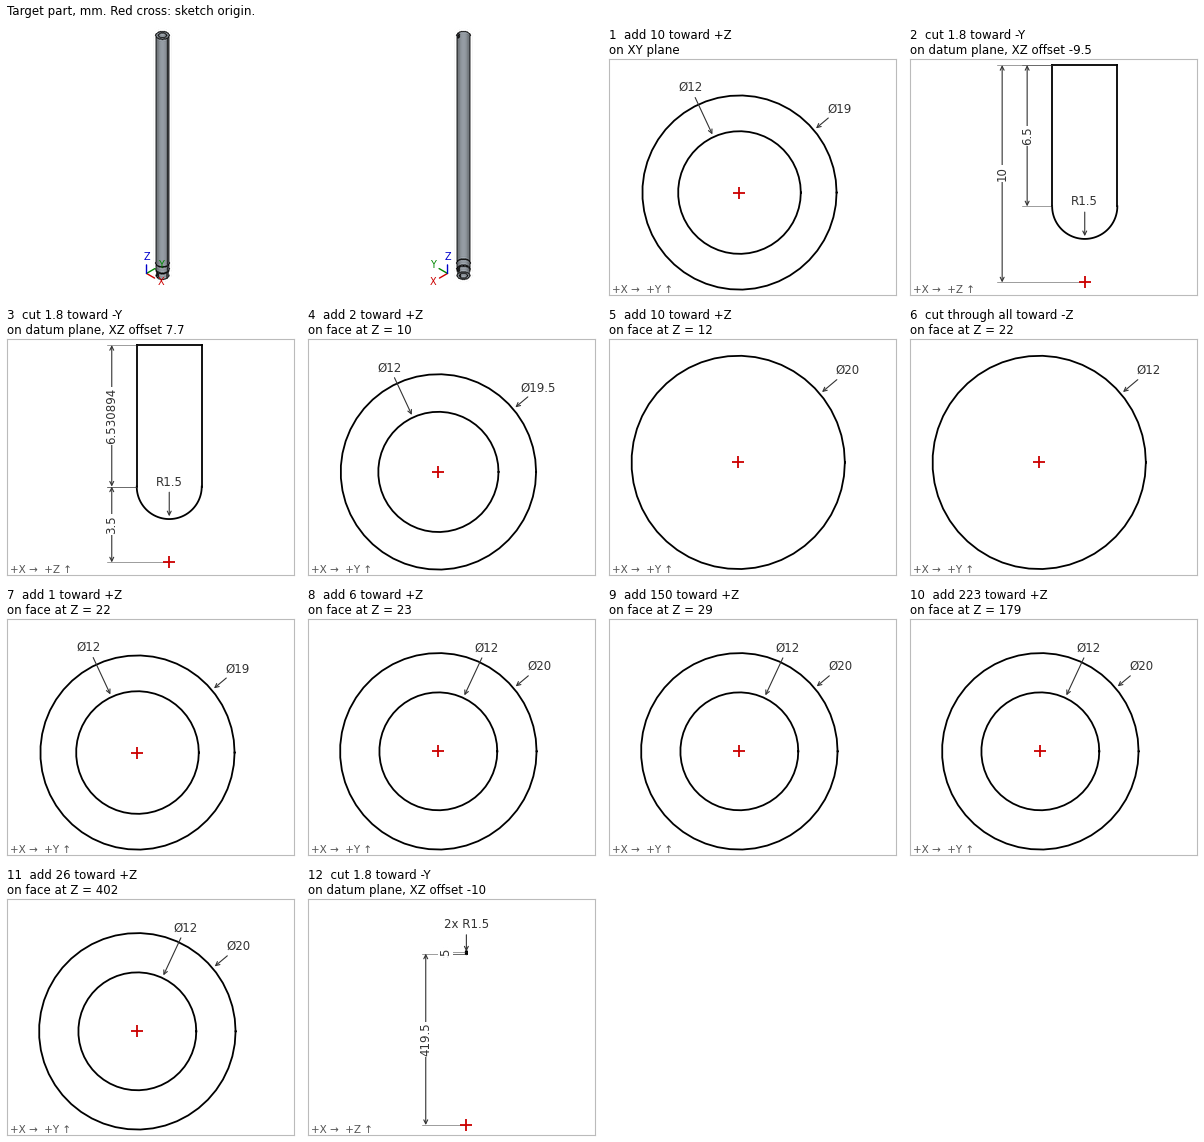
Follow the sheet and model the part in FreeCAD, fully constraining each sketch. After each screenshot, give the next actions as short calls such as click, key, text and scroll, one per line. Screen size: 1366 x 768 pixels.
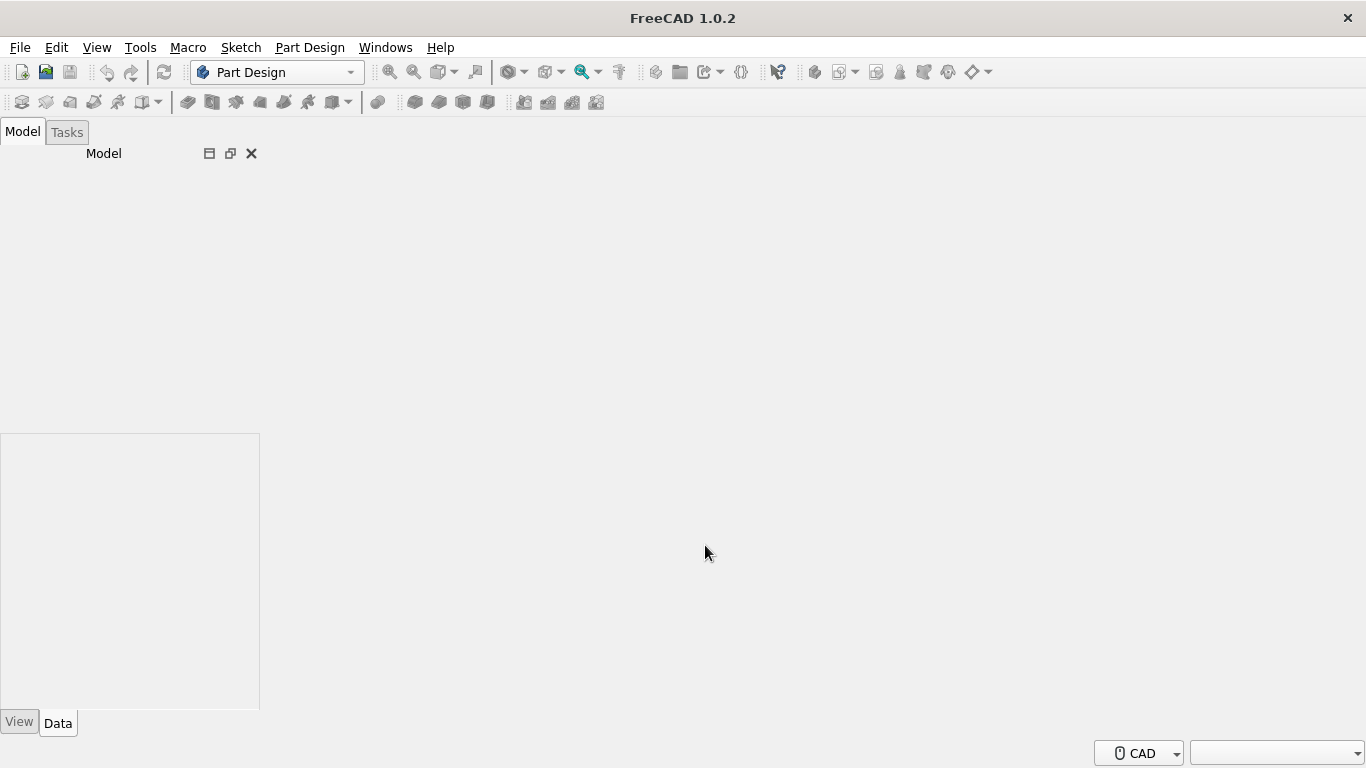
click(22, 72)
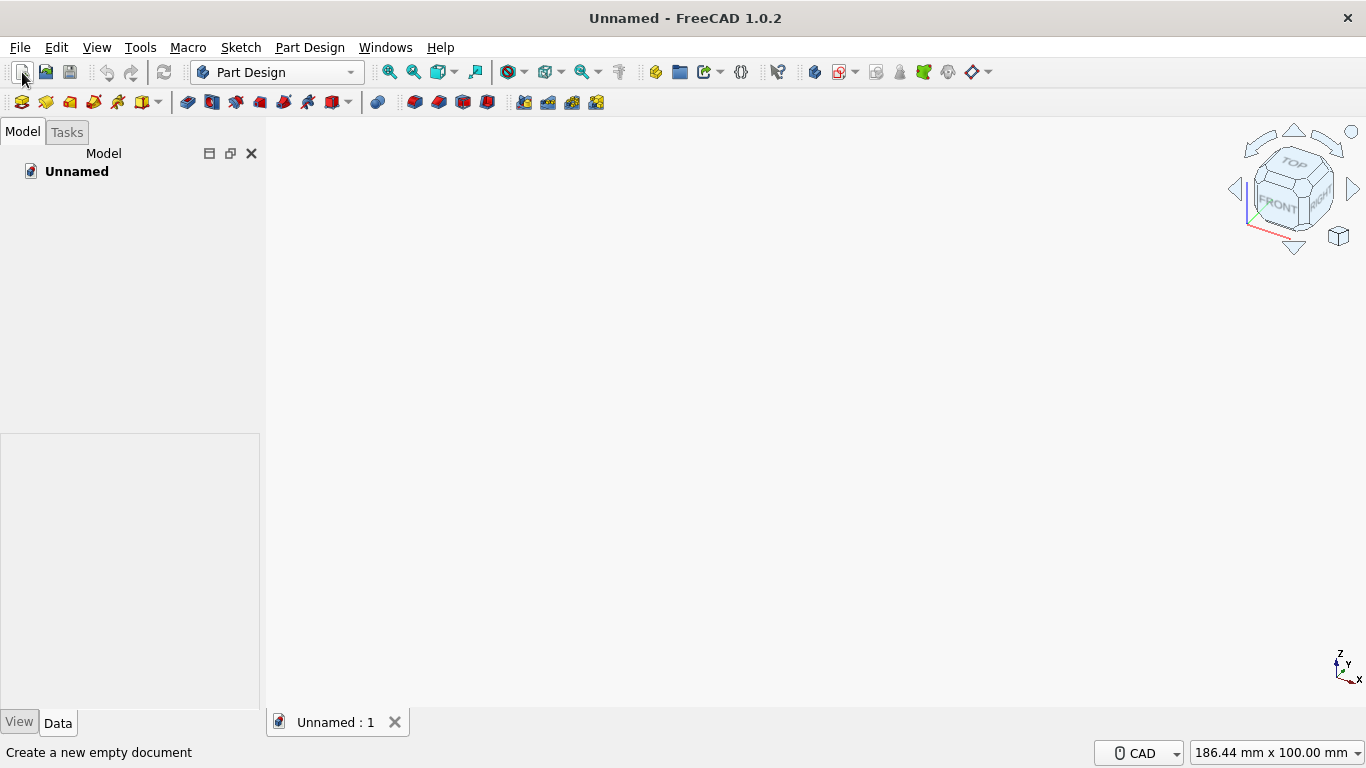
click(840, 72)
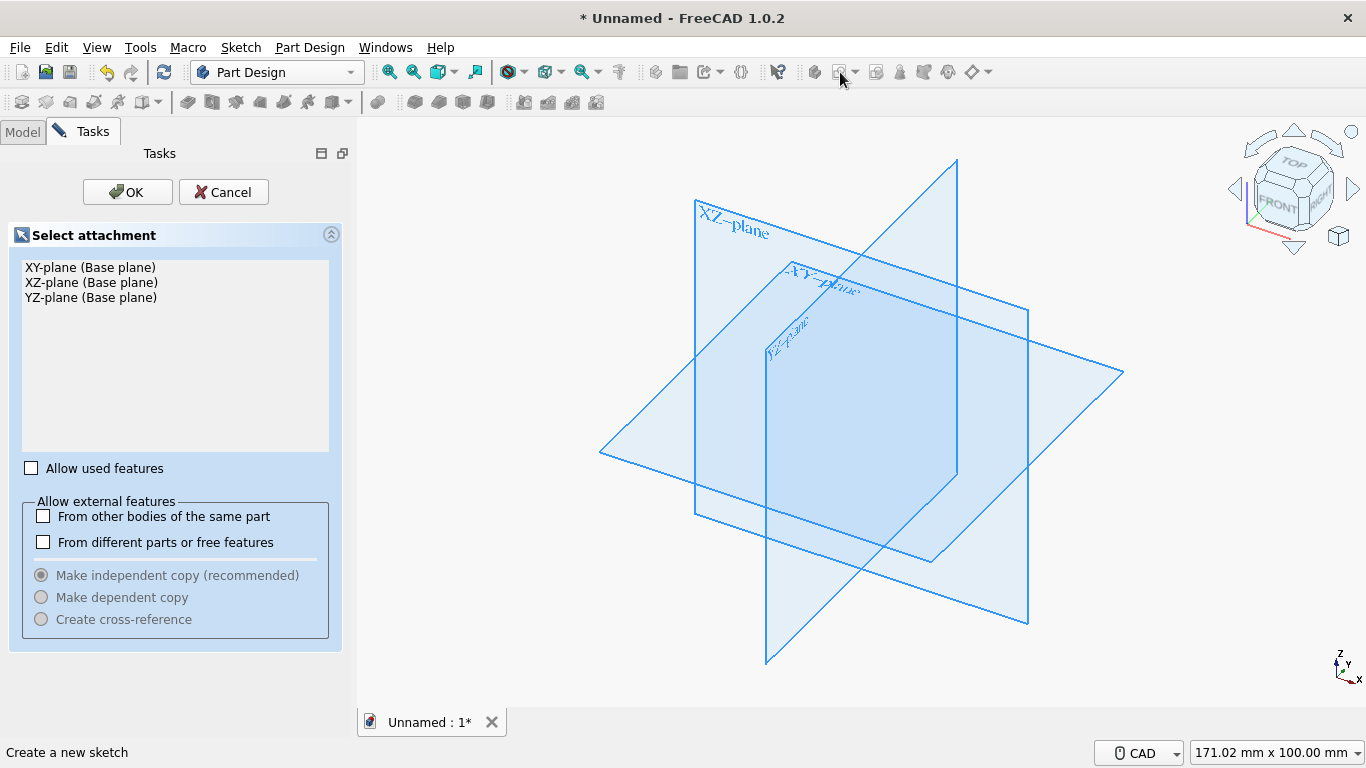
click(82, 268)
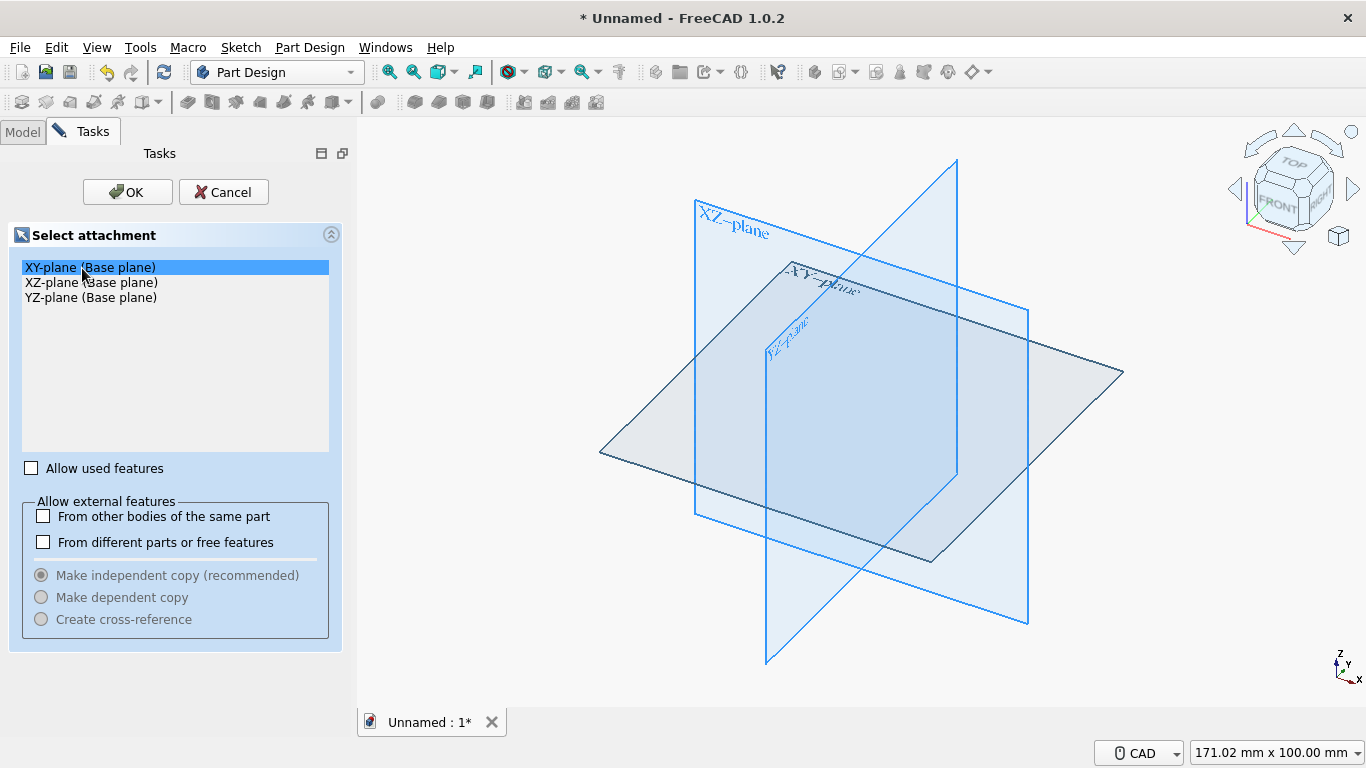
click(128, 192)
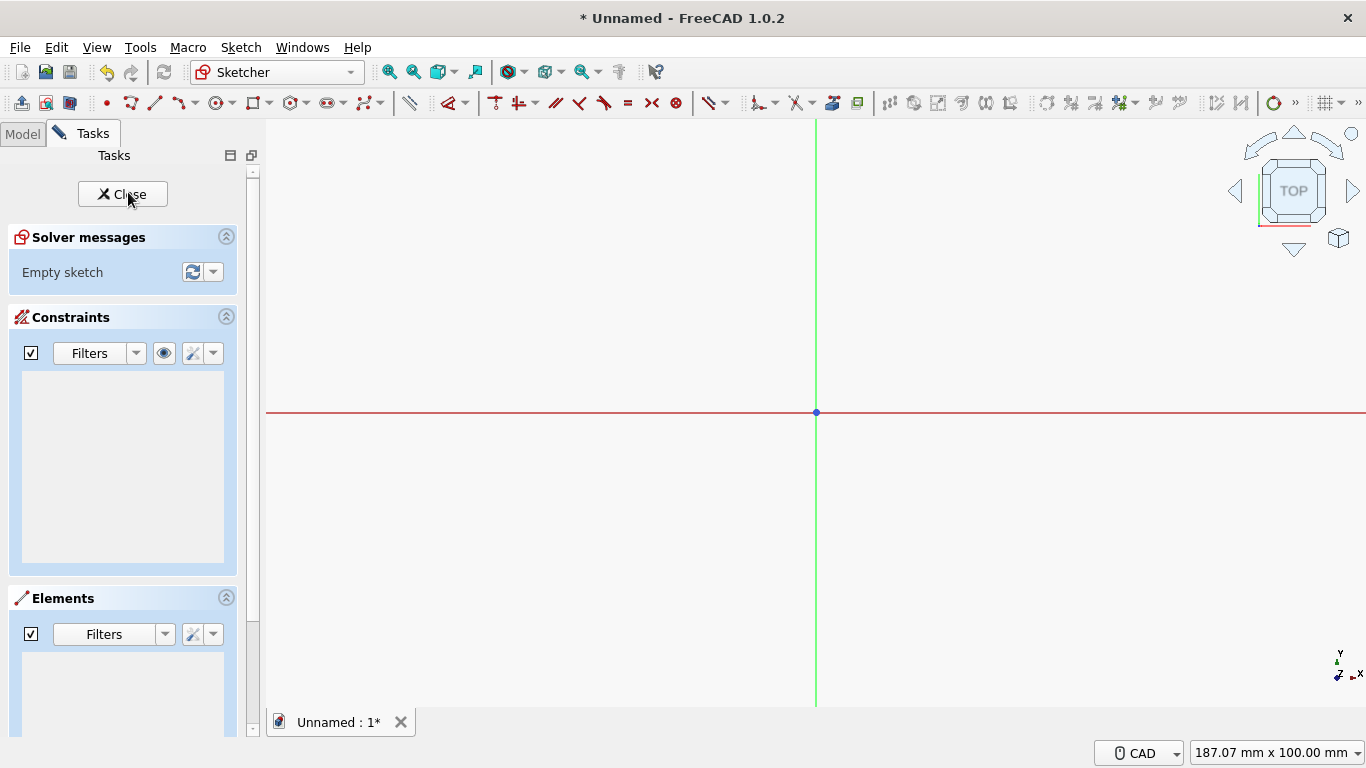
scroll(846, 413, up, 6)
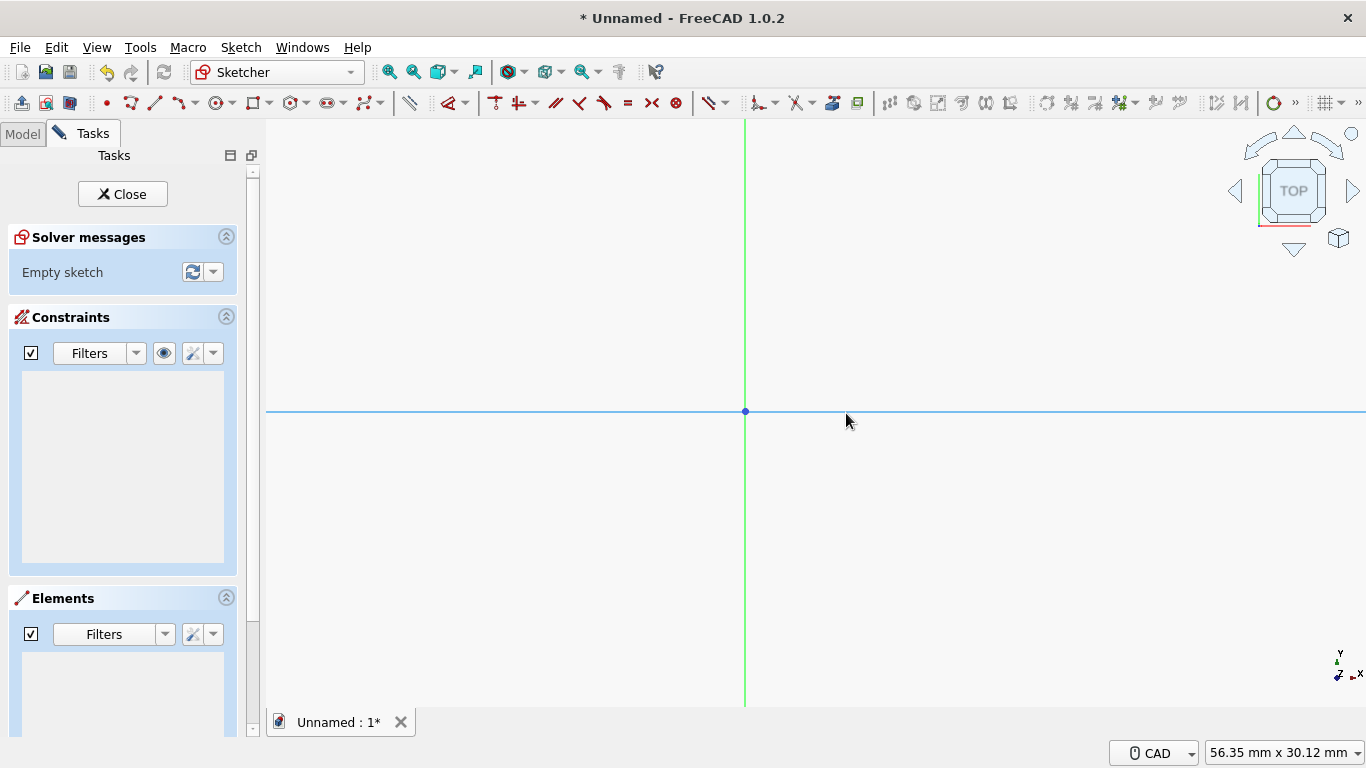
click(216, 104)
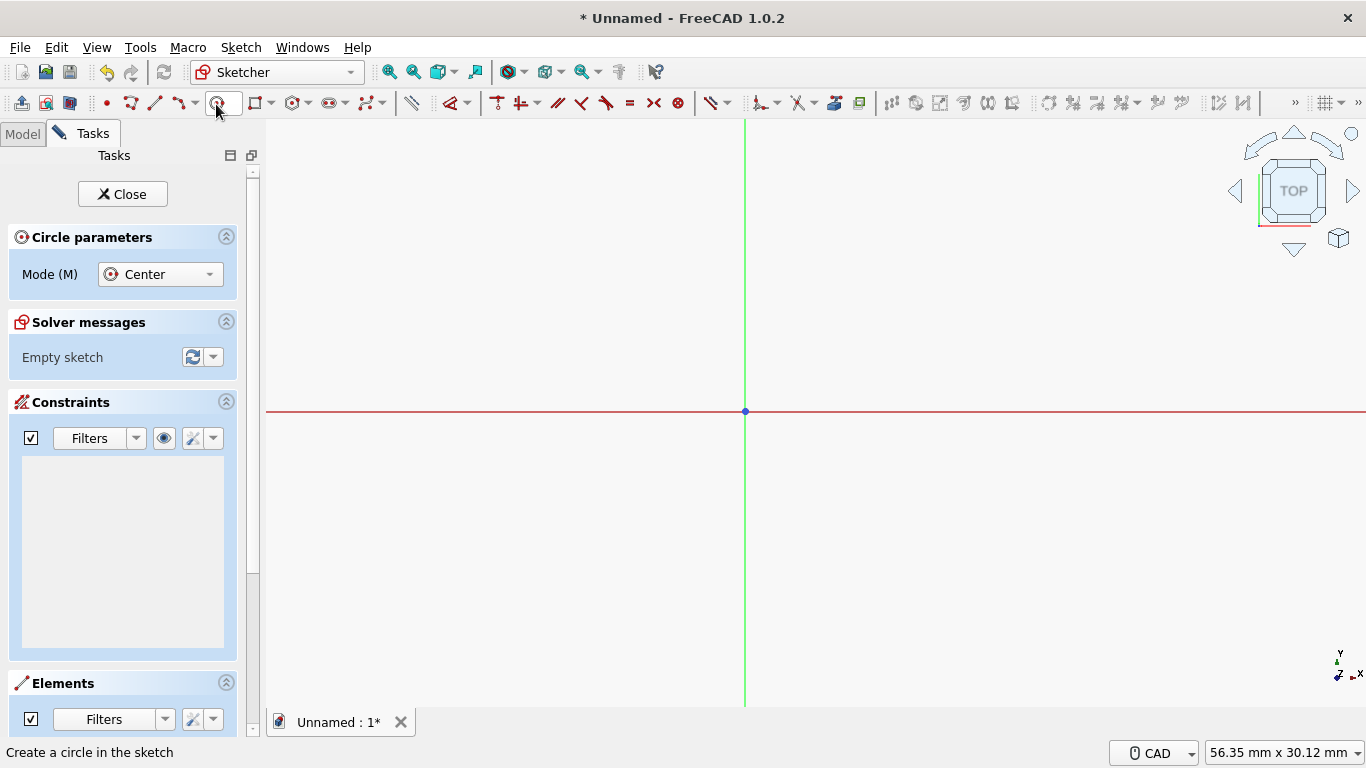
click(745, 412)
click(876, 281)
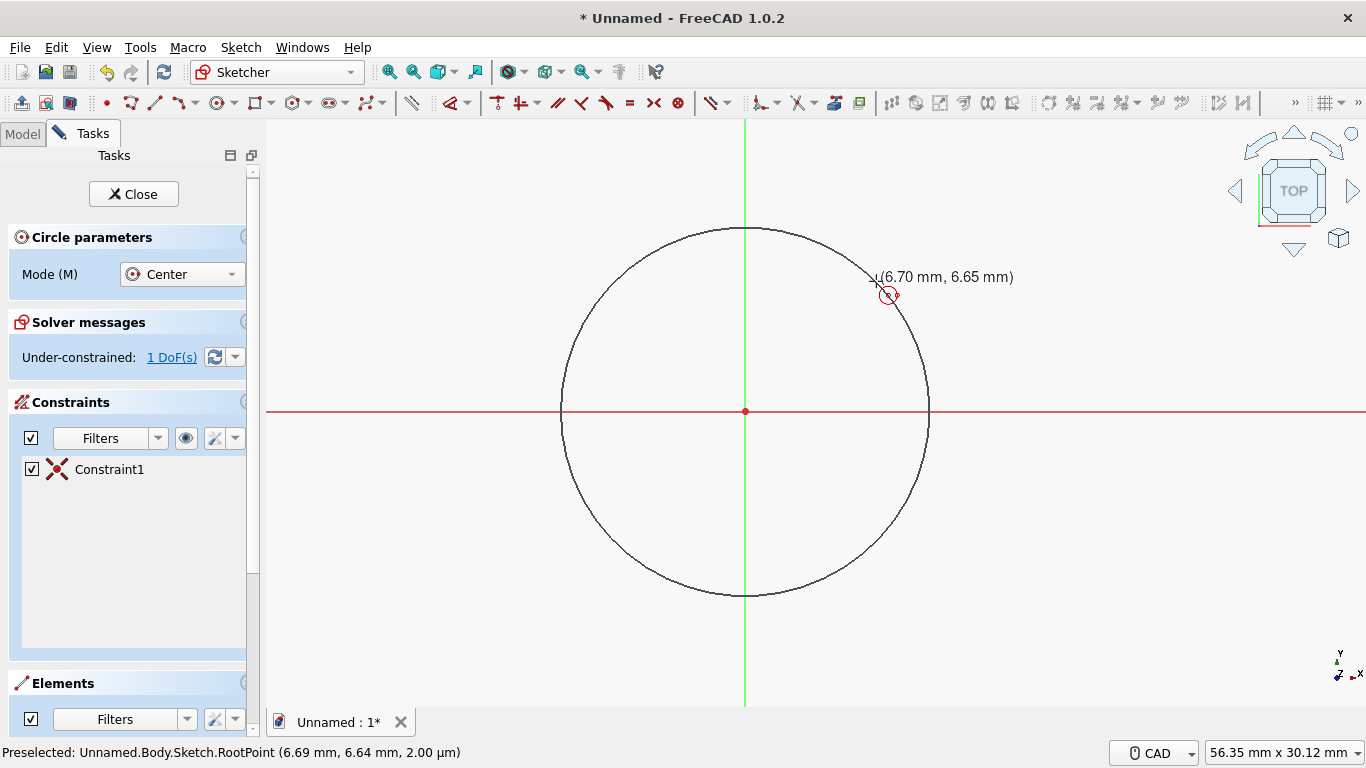
click(745, 412)
click(828, 329)
key(Escape)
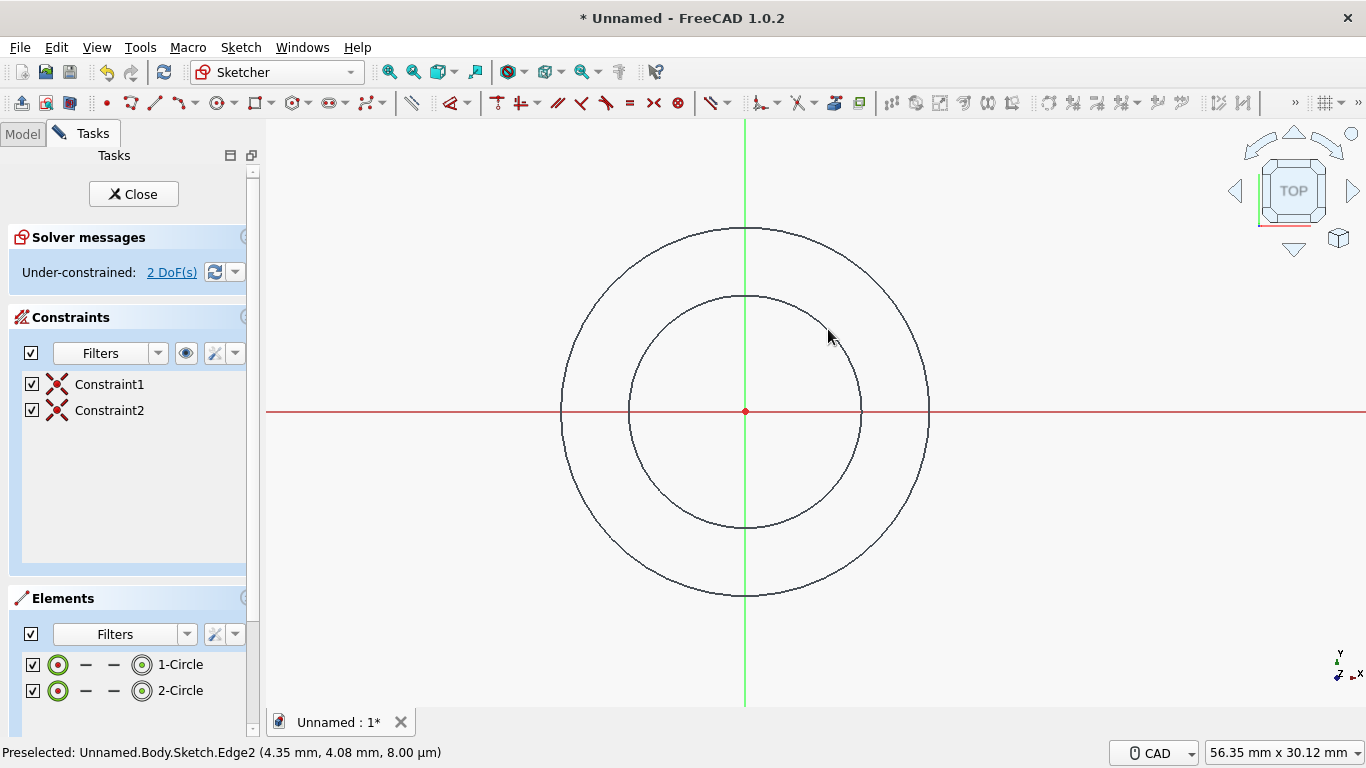
click(450, 104)